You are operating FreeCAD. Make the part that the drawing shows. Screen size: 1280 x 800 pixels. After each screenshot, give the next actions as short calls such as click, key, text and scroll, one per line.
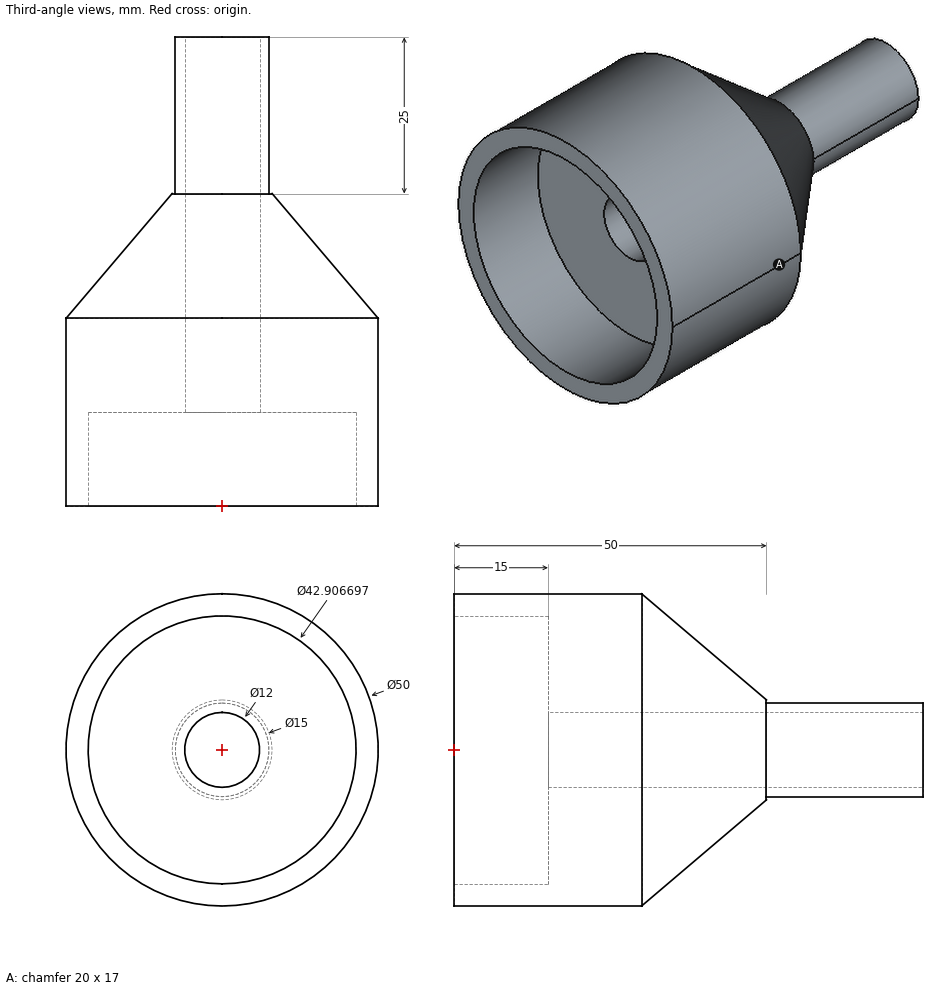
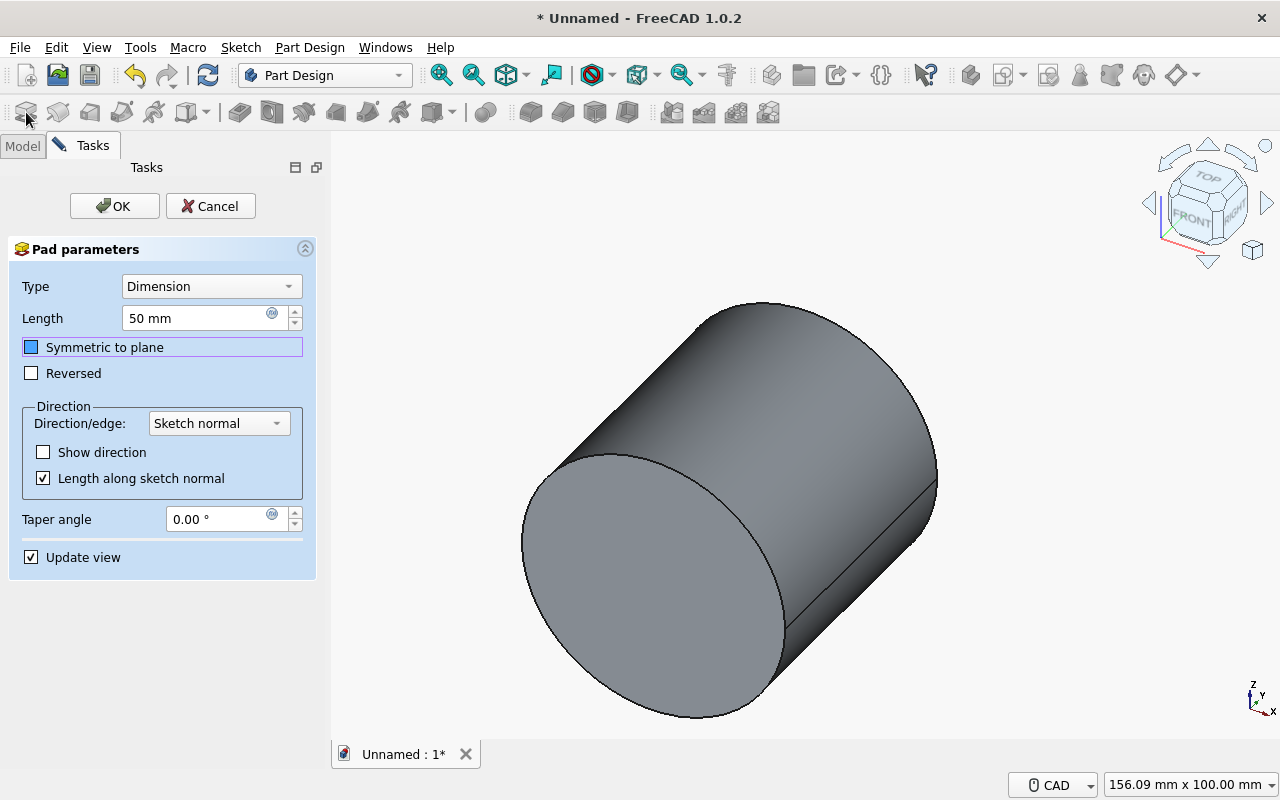
click(30, 373)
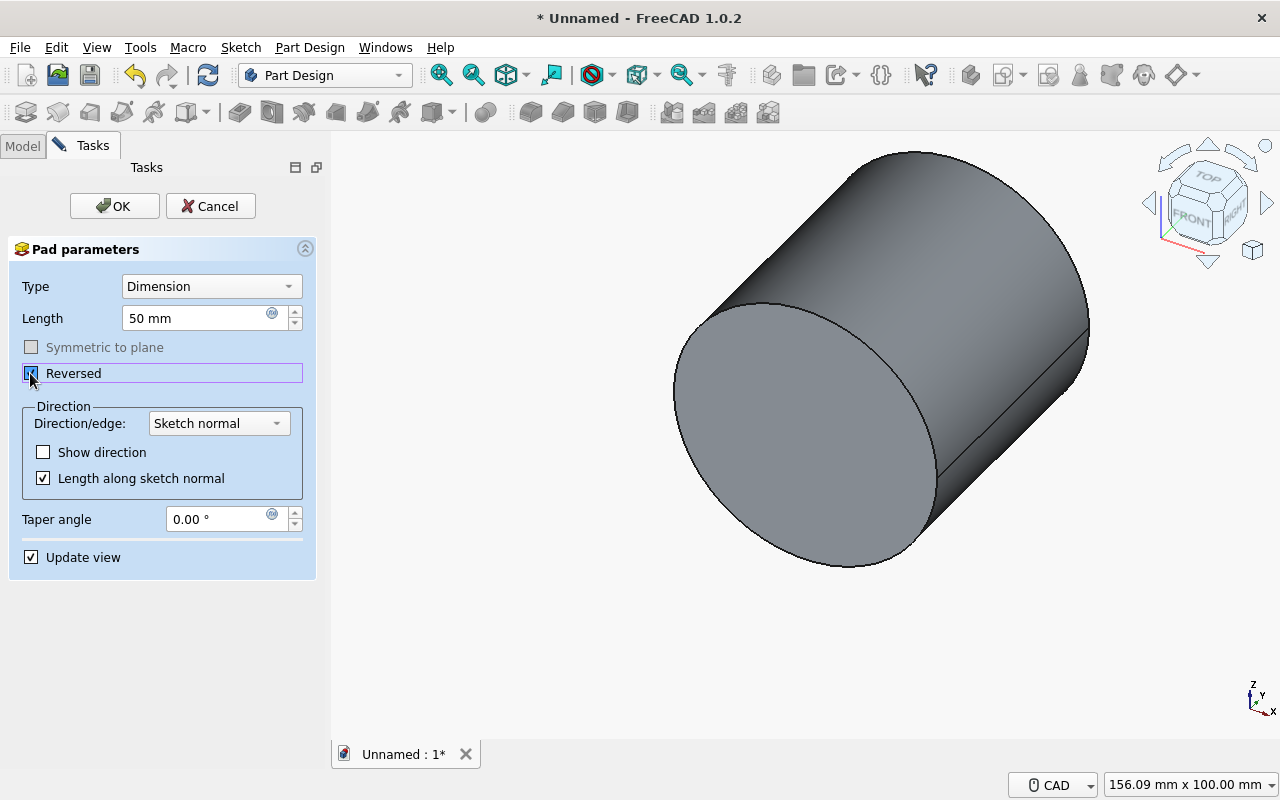
click(115, 206)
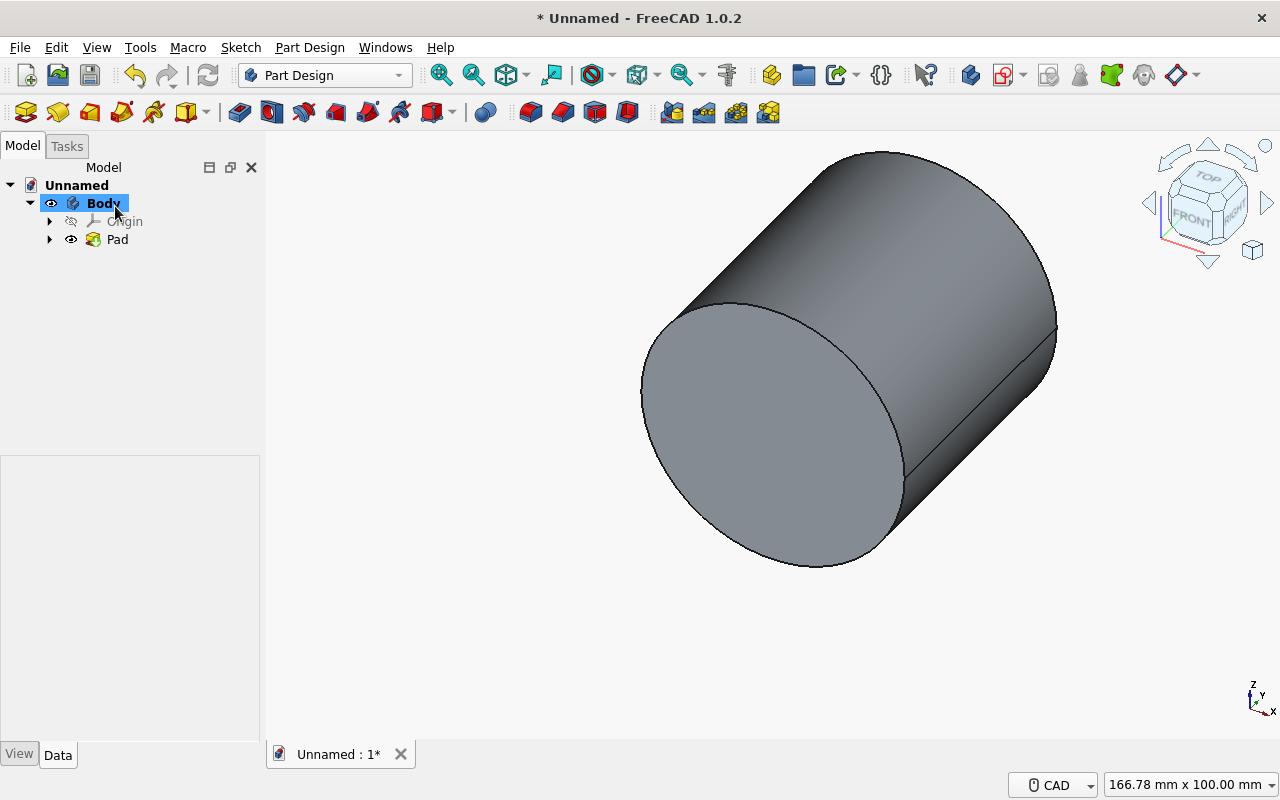
click(442, 76)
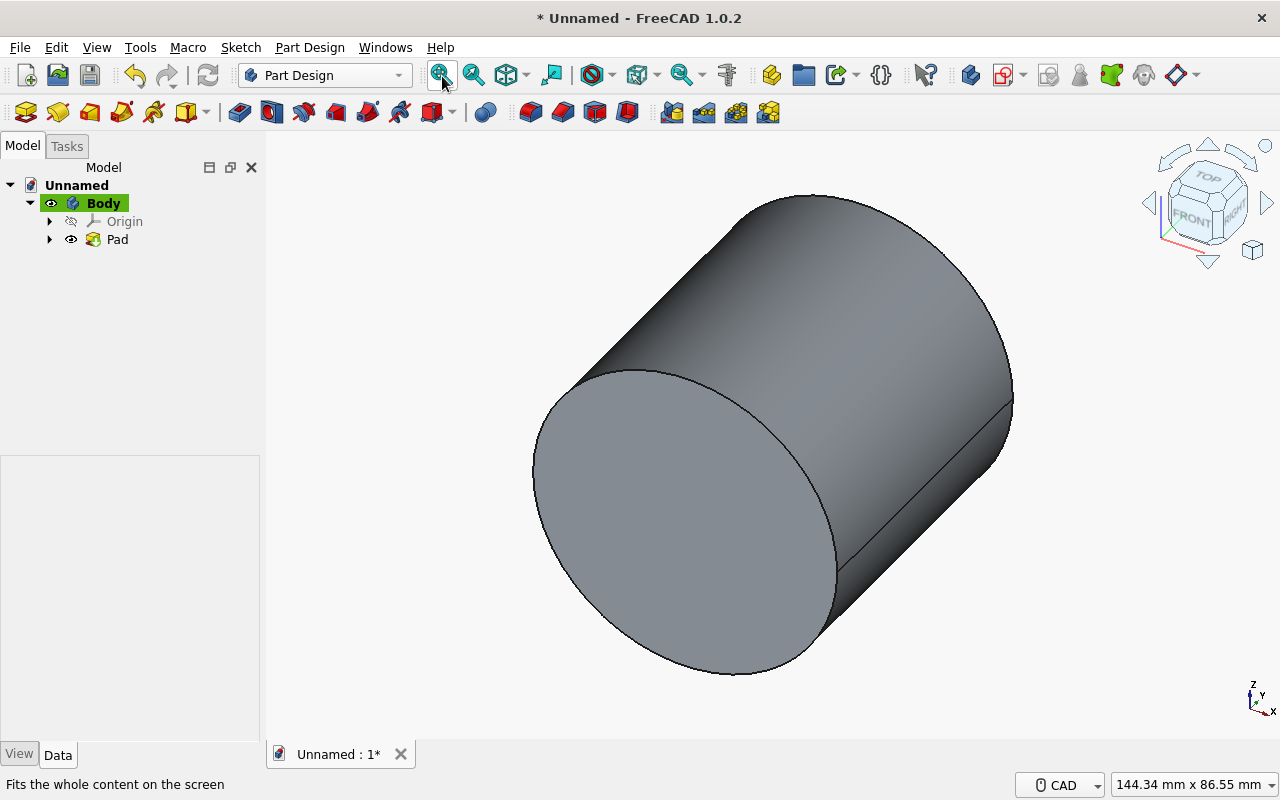
key(4)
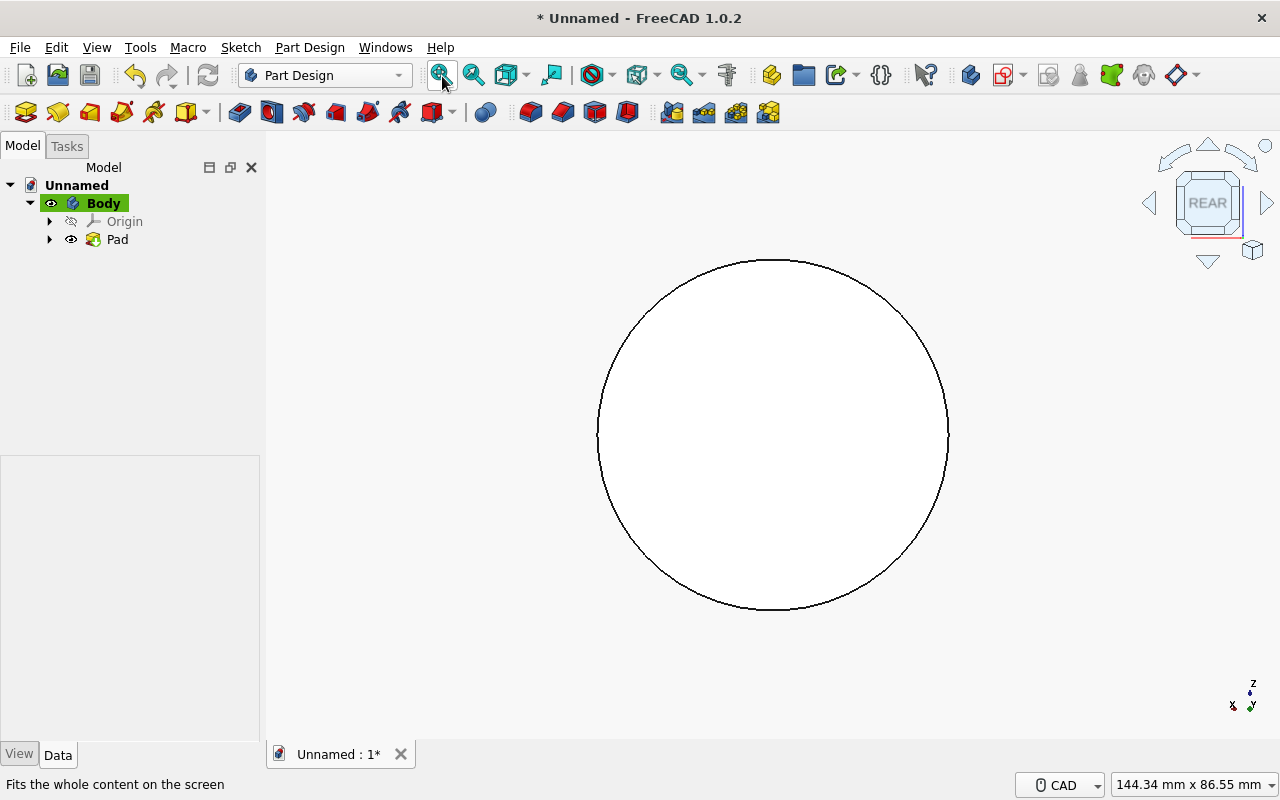
click(773, 434)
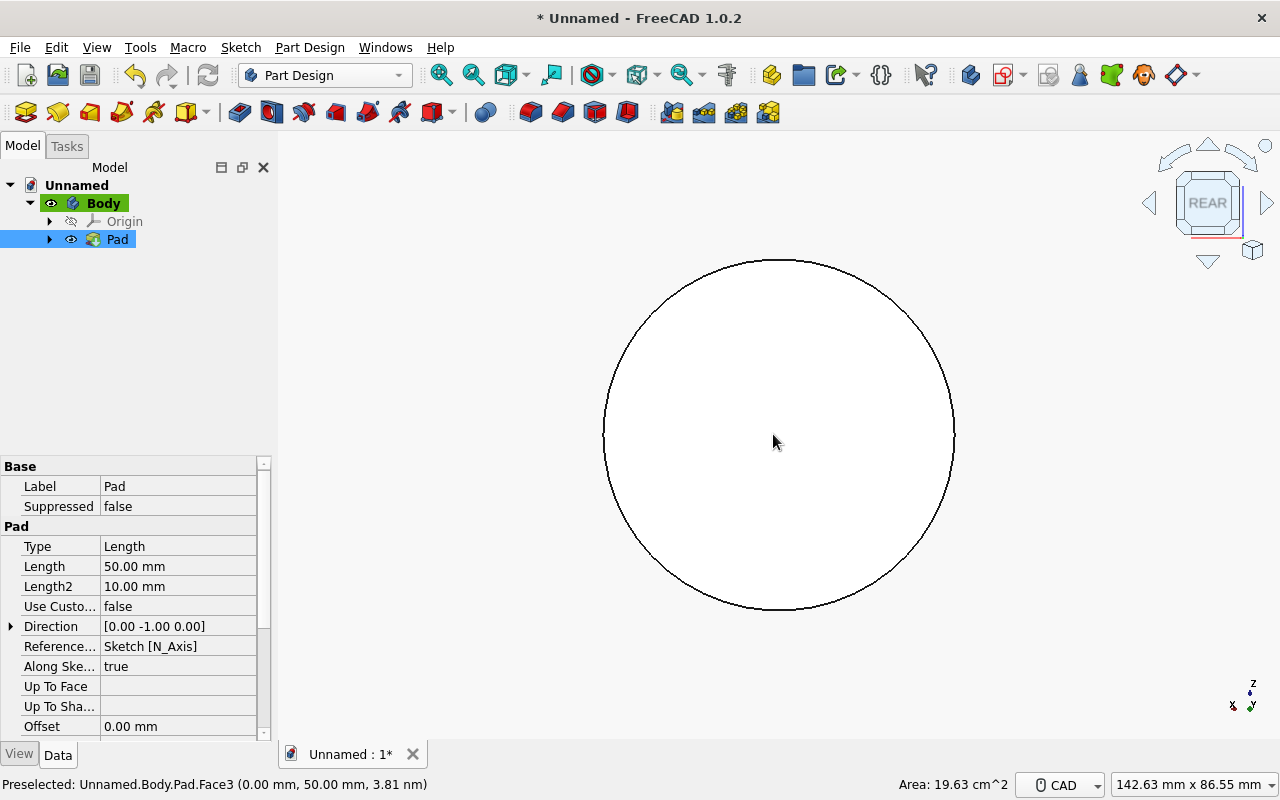
click(1004, 76)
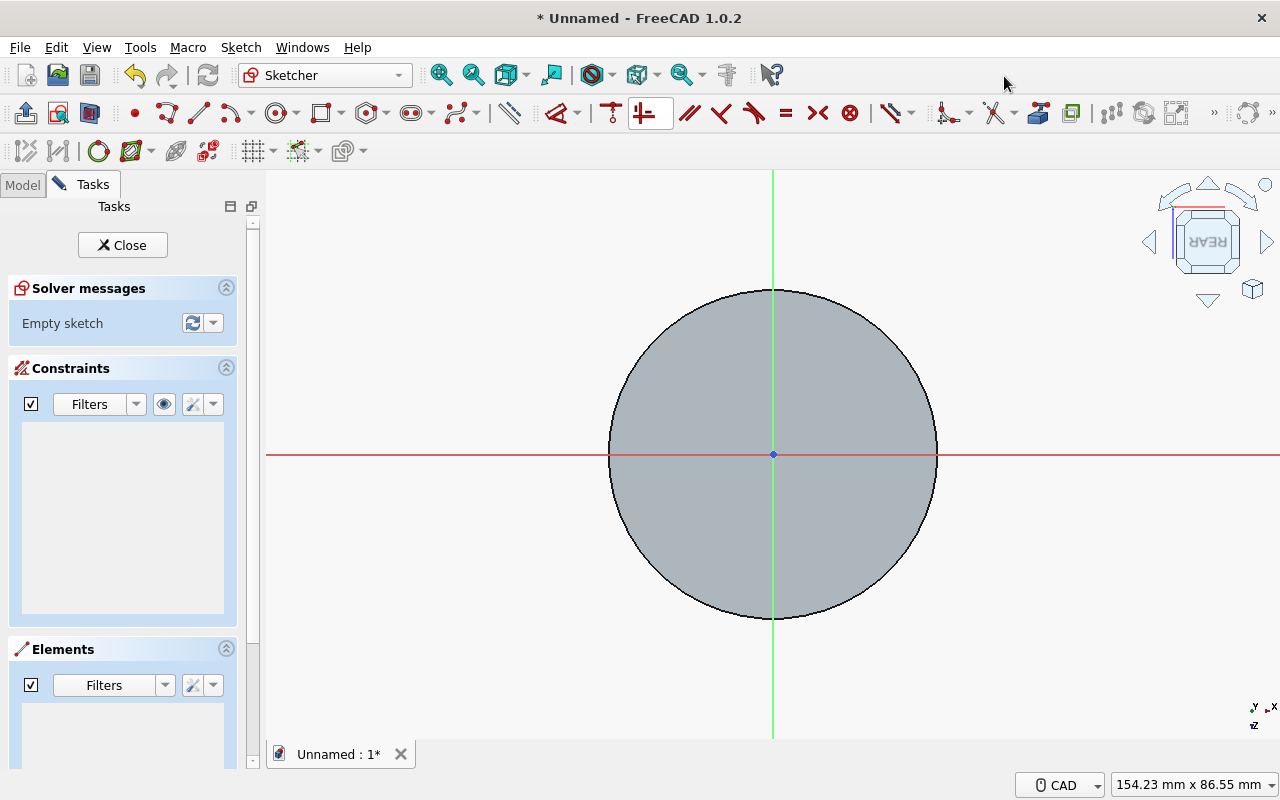
scroll(795, 454, up, 7)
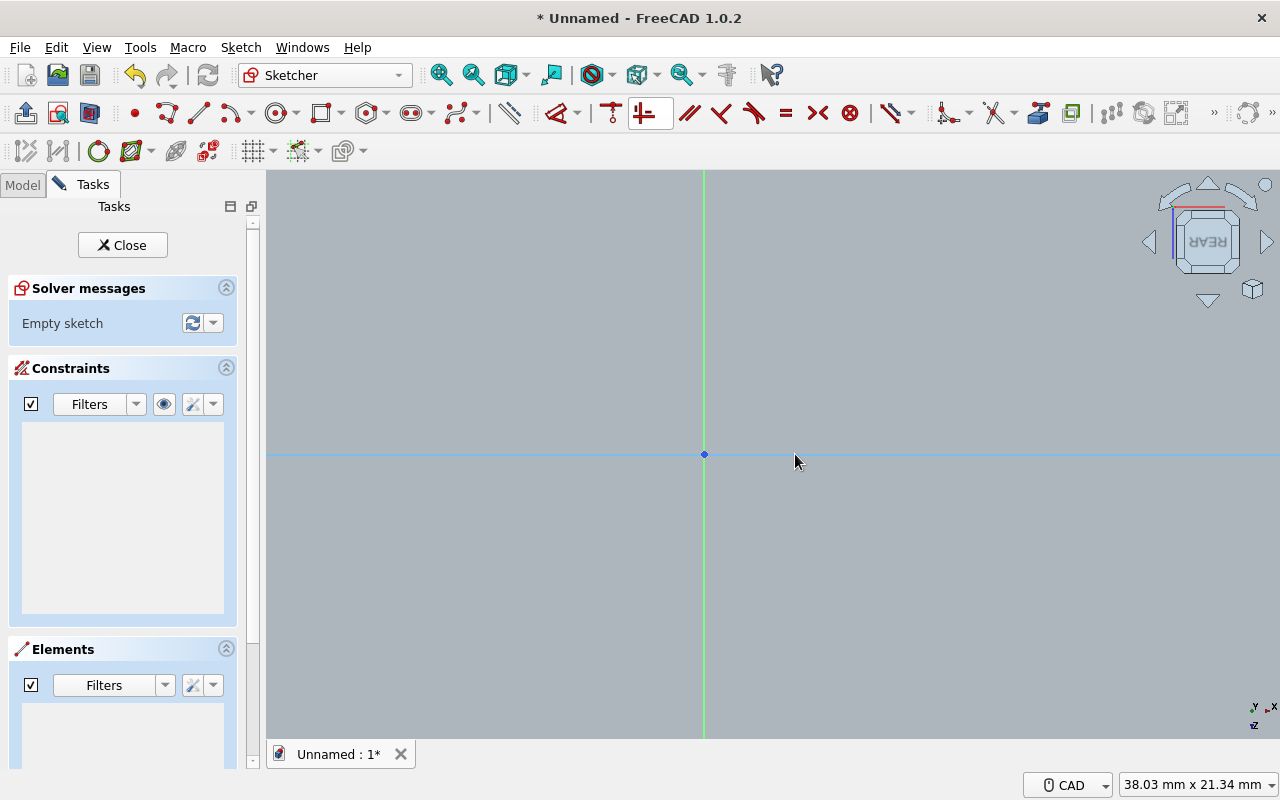
click(276, 114)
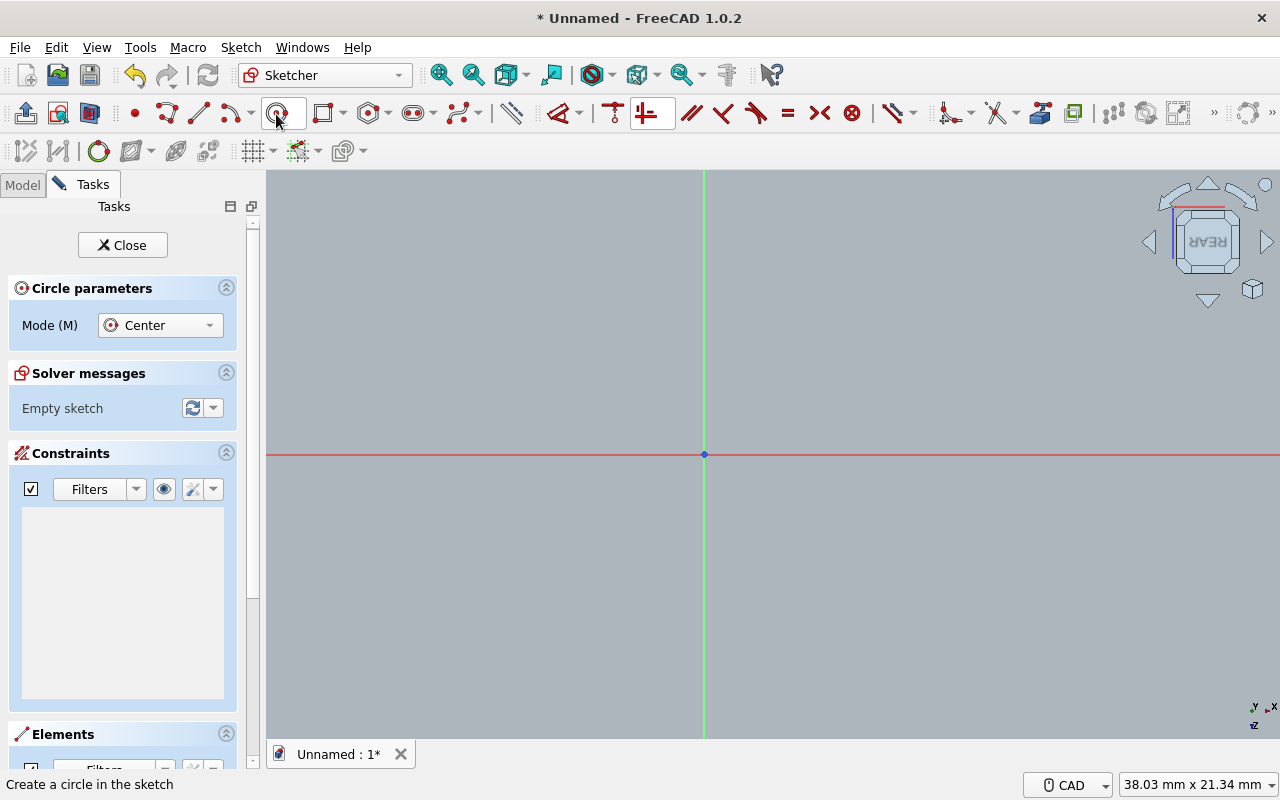
click(704, 454)
move(846, 313)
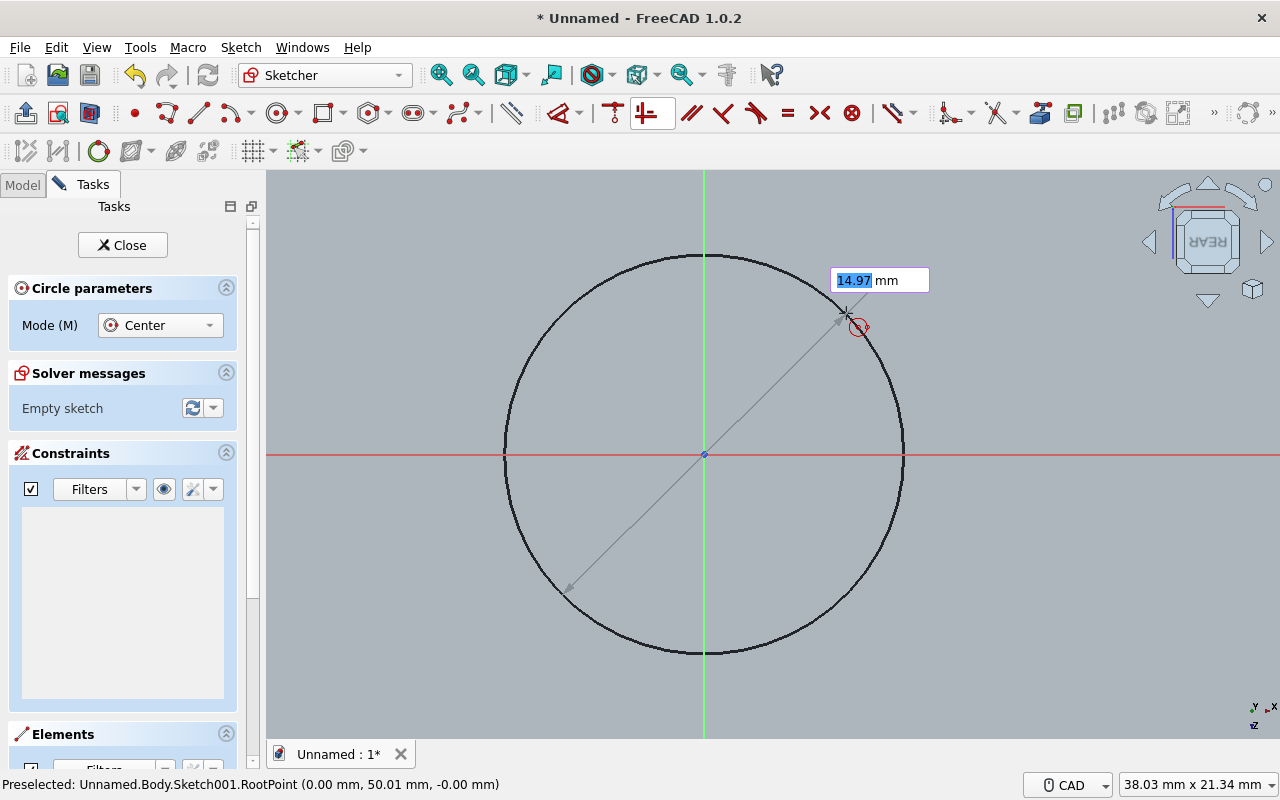
text(15)
key(Return)
key(Escape)